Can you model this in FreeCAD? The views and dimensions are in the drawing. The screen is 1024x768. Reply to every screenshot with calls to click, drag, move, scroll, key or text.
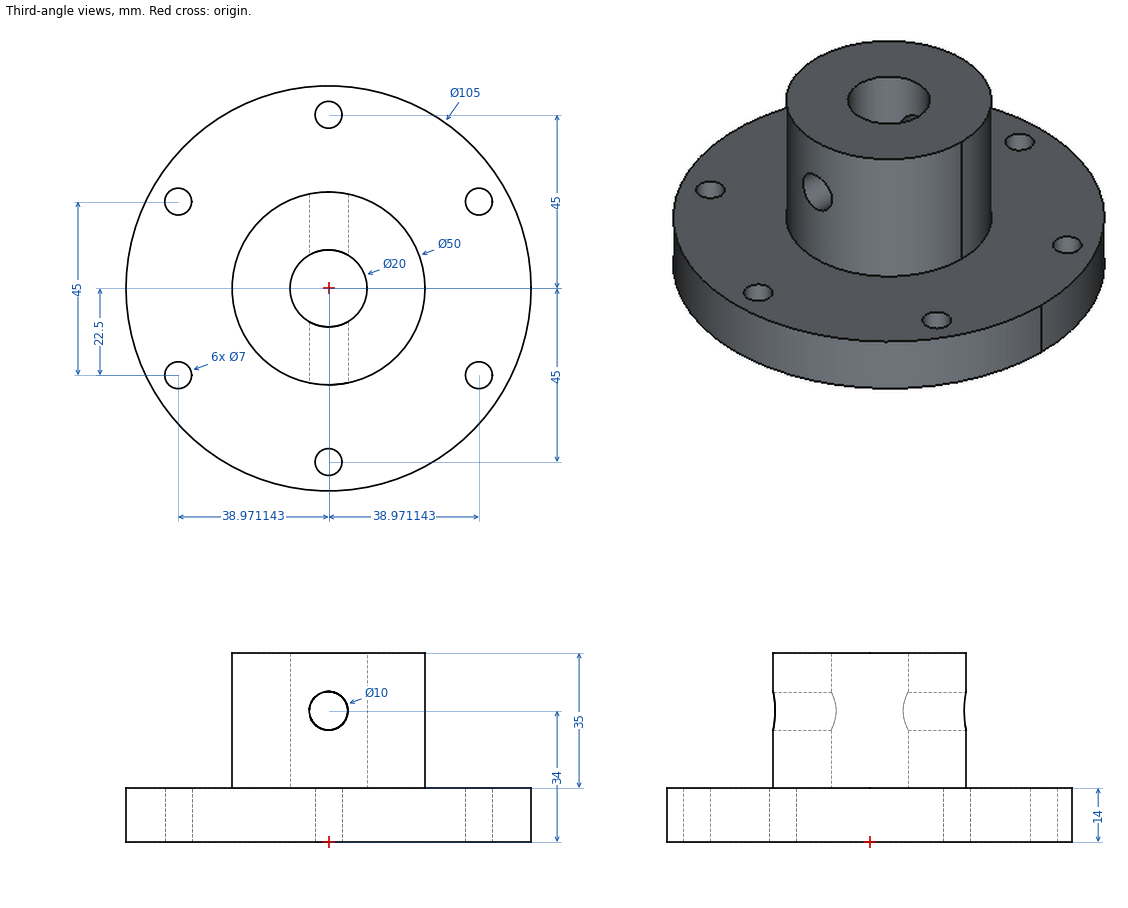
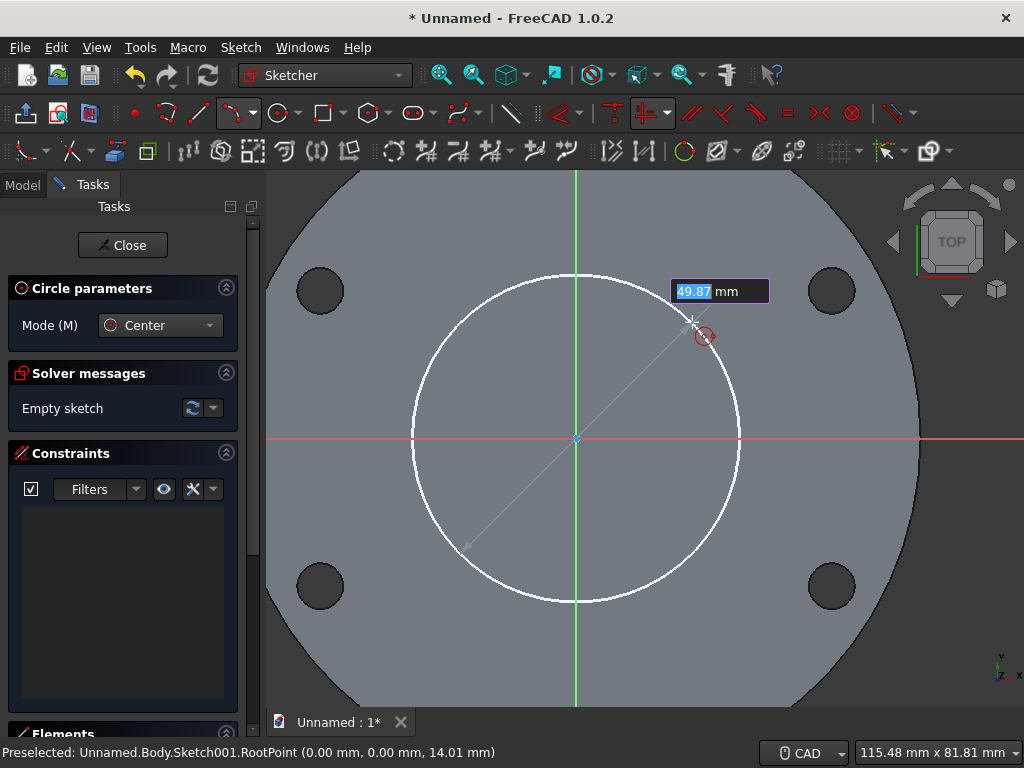
text(50)
key(Return)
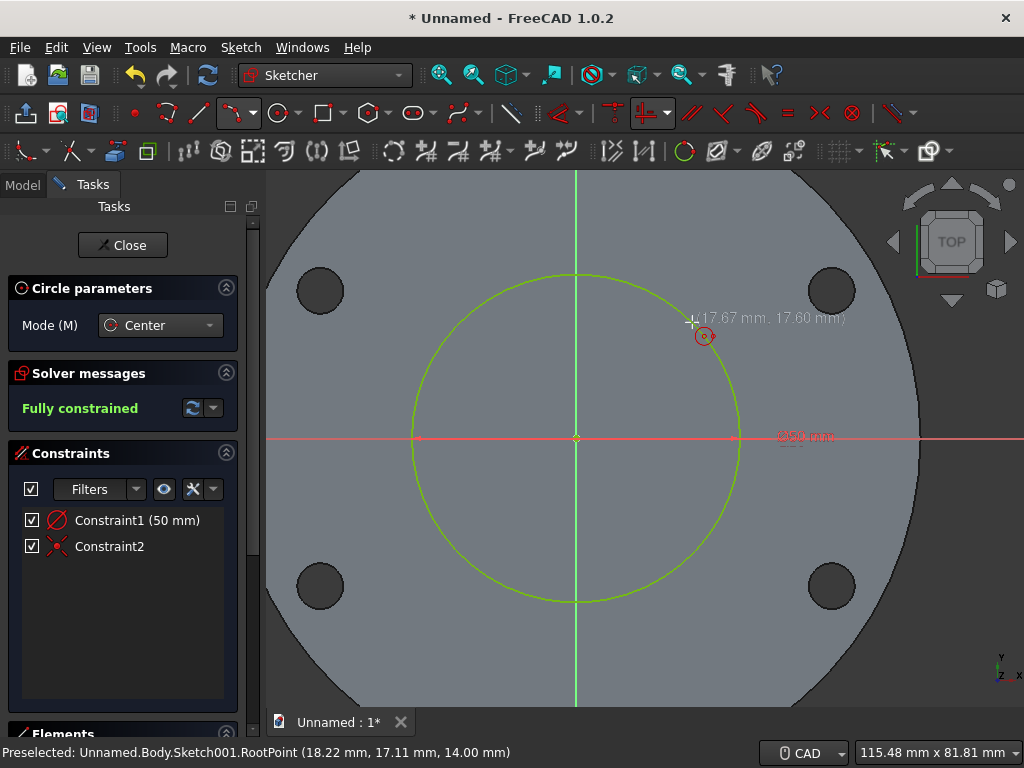
click(576, 438)
move(622, 392)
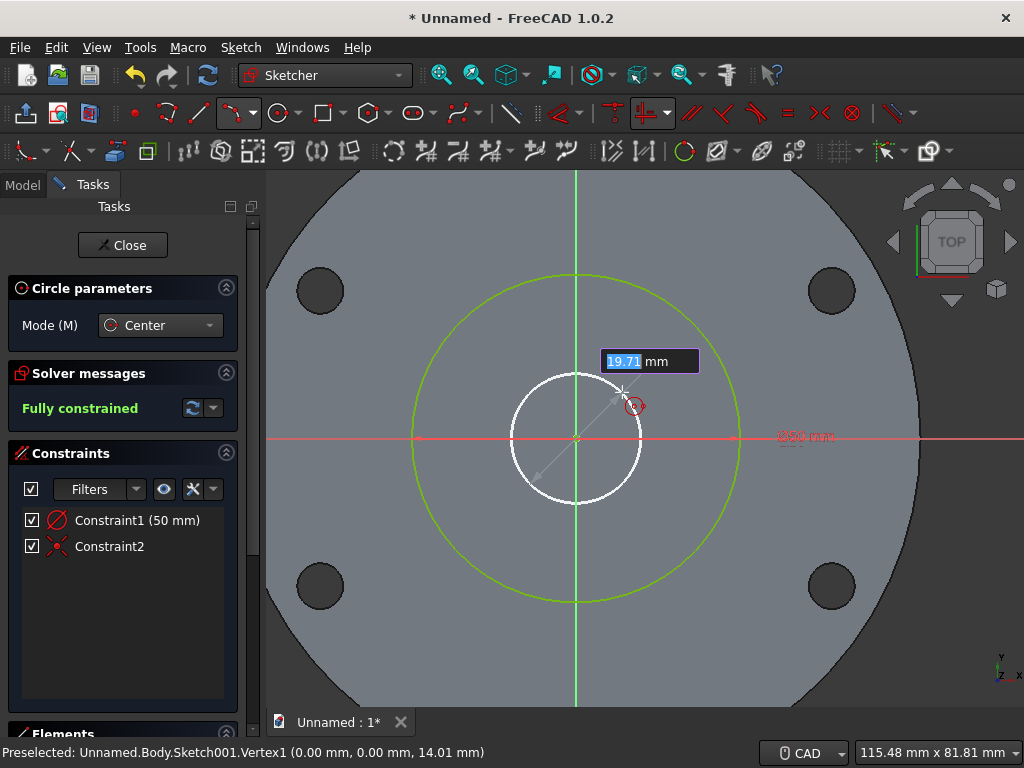
text(20)
key(Return)
key(Escape)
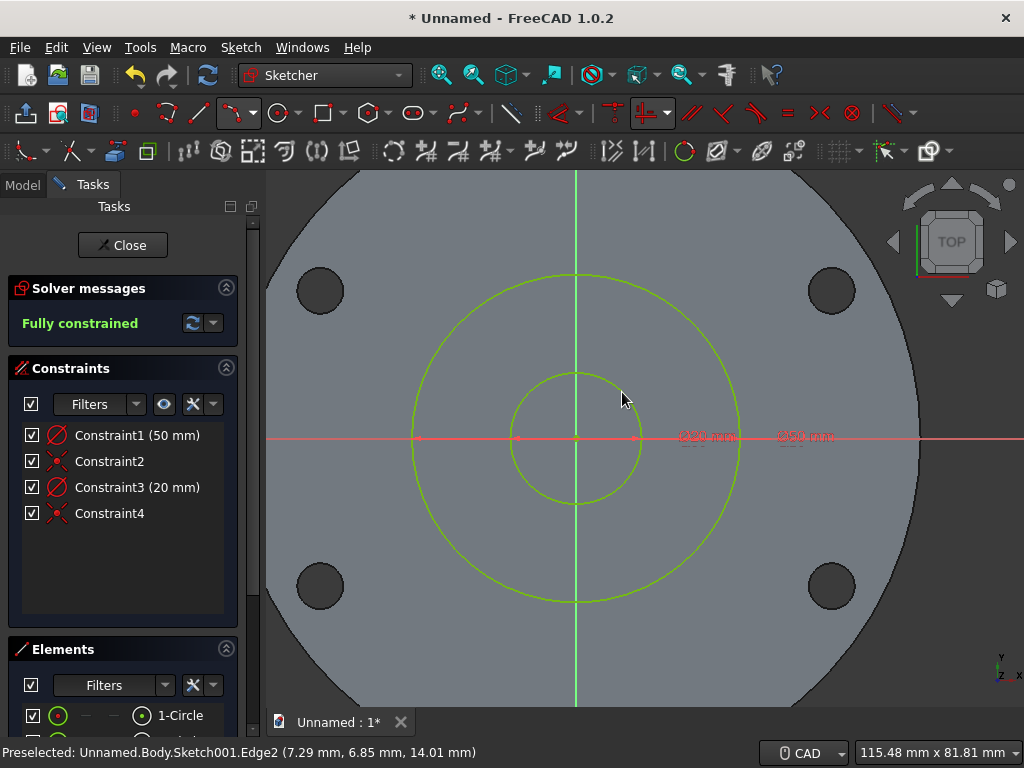
click(123, 245)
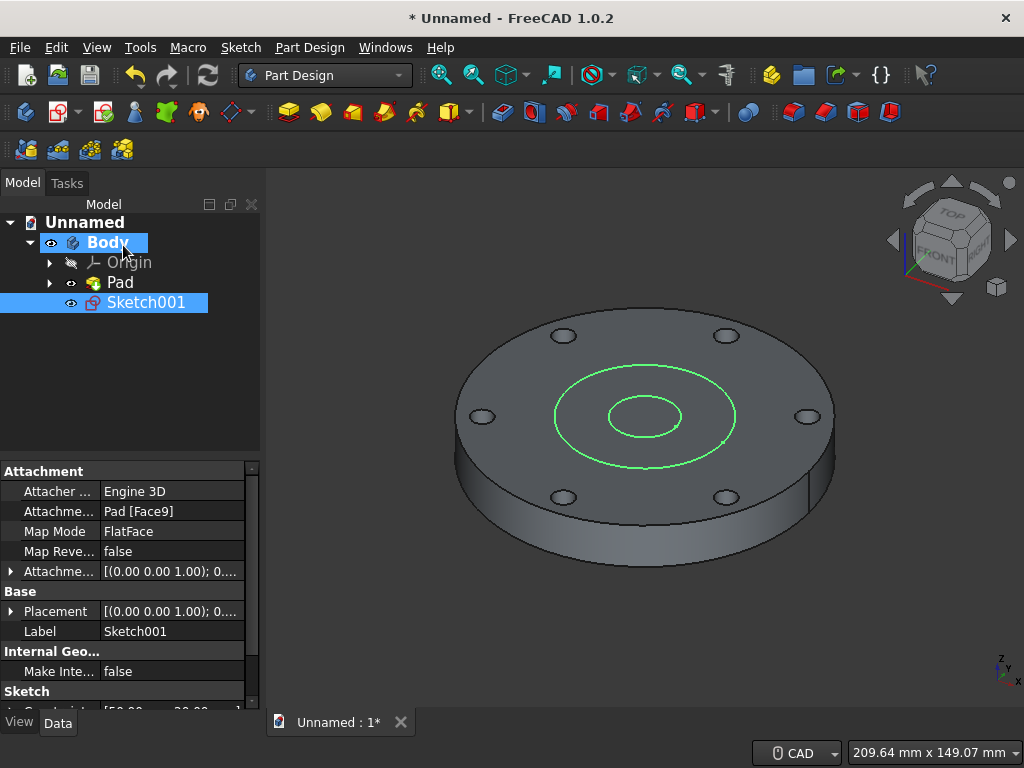
click(290, 112)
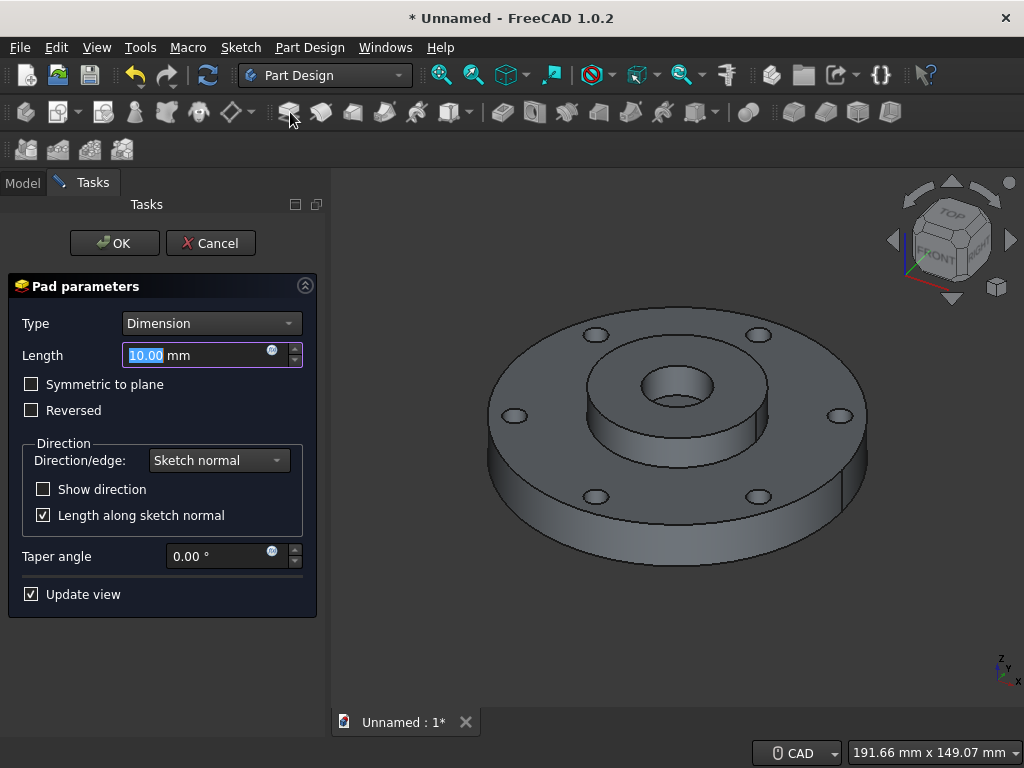
text(35)
key(Tab)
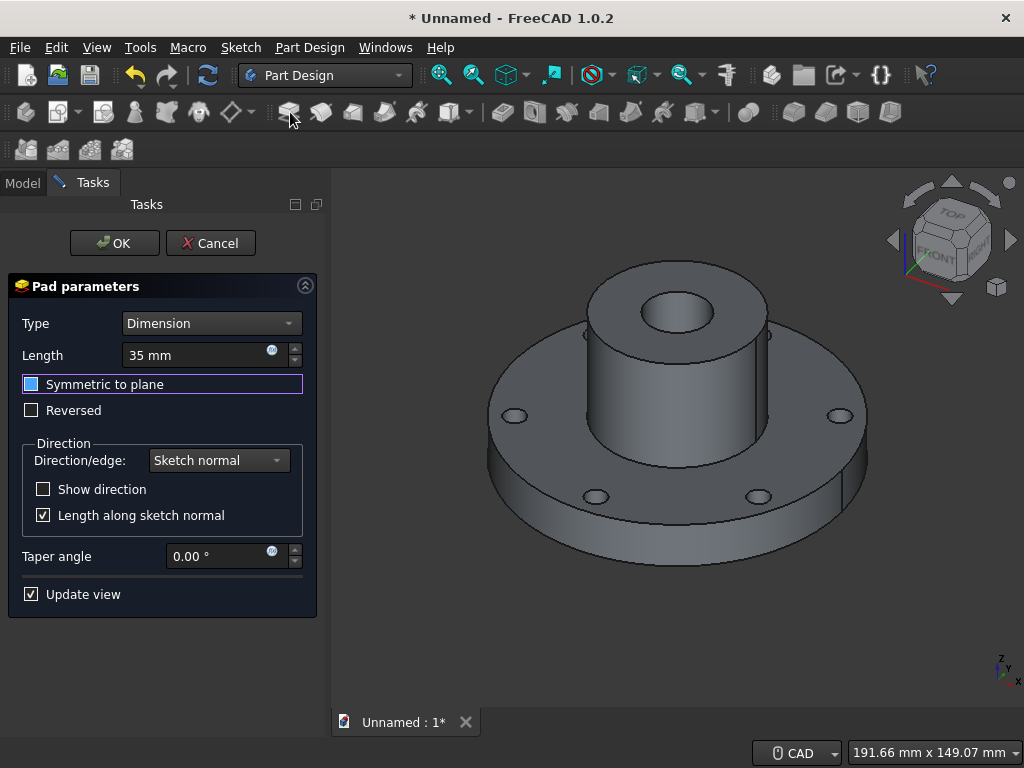
click(115, 243)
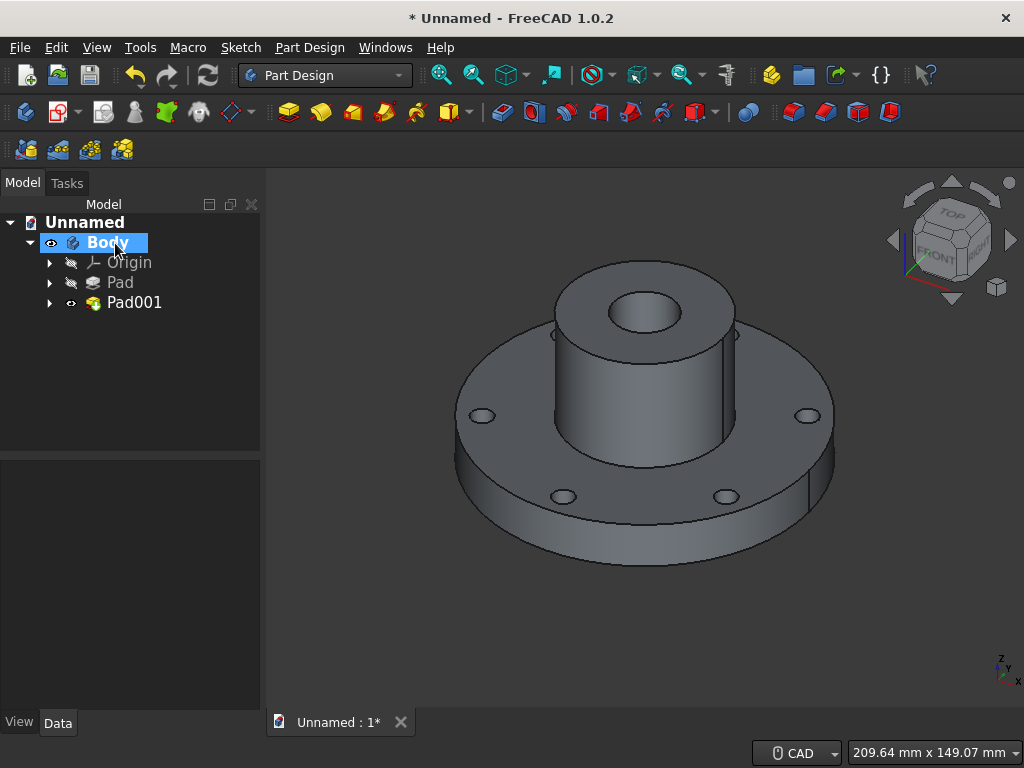
click(442, 76)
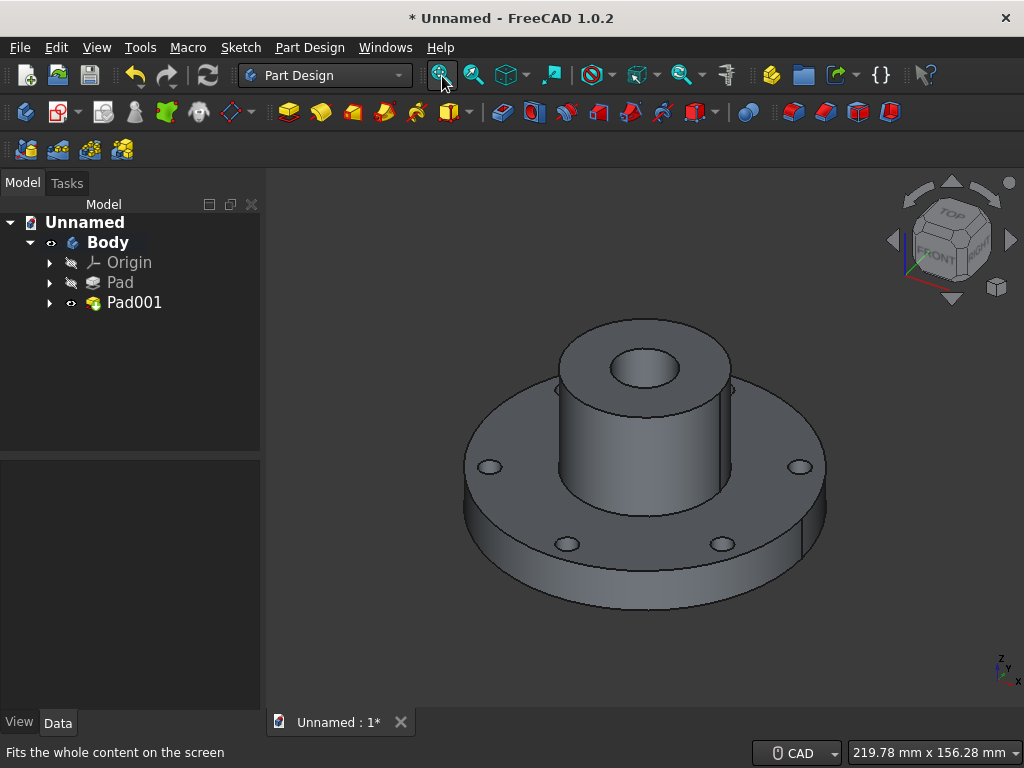
click(58, 112)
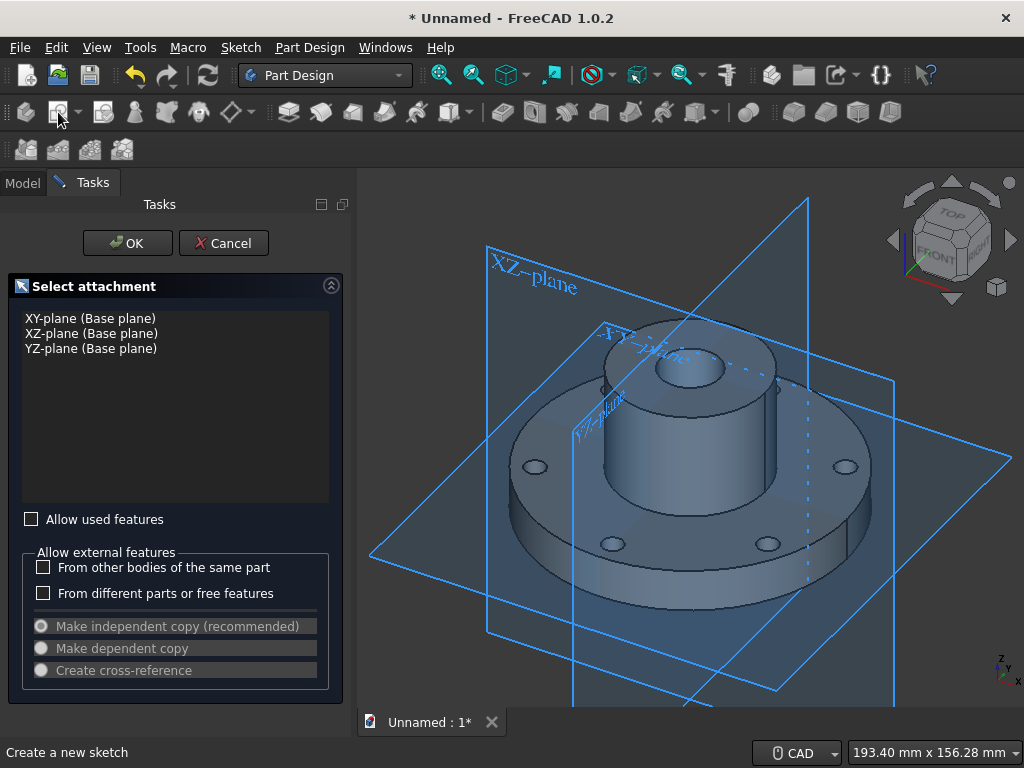
click(82, 334)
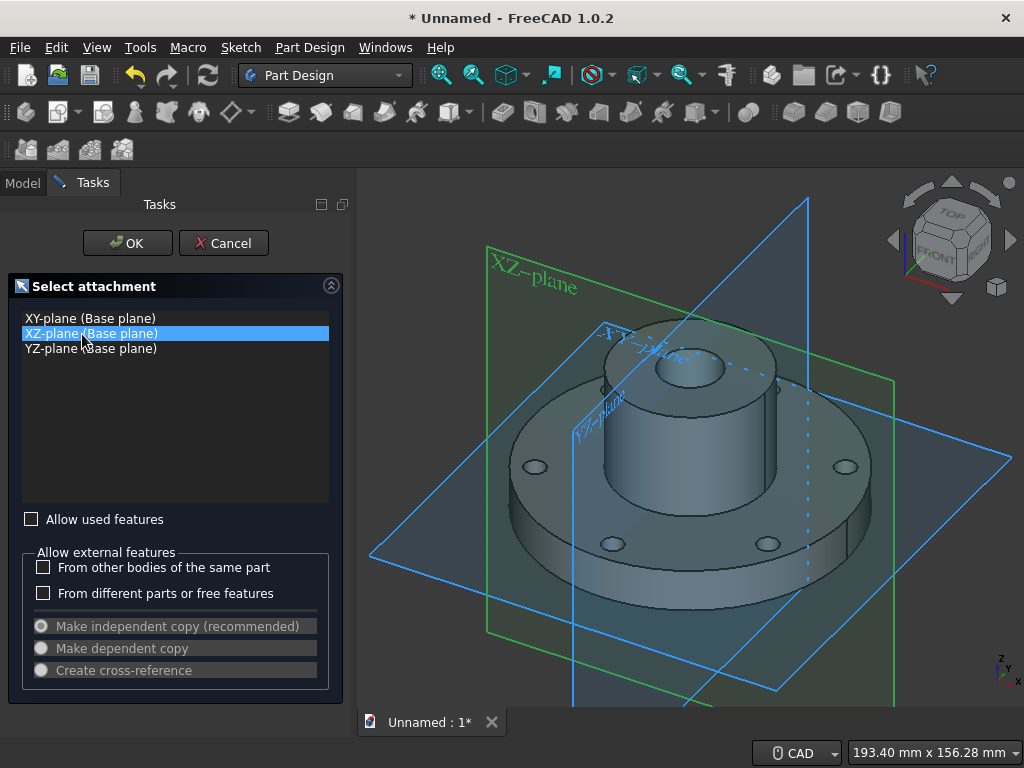
click(128, 243)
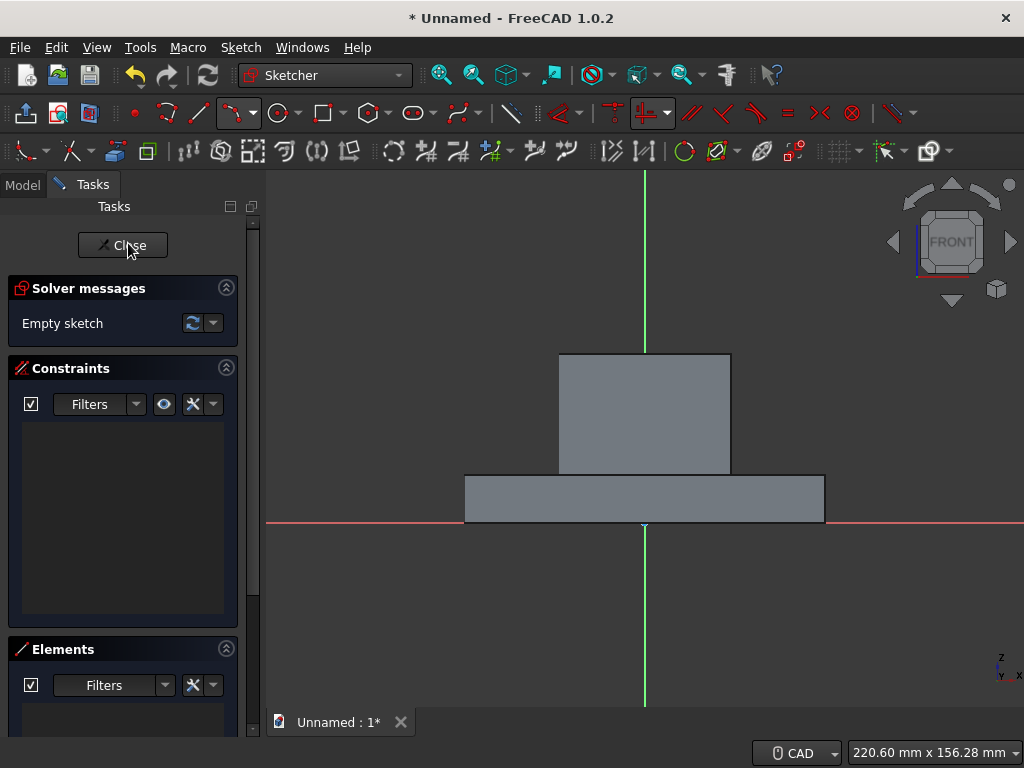
key(q)
key(s)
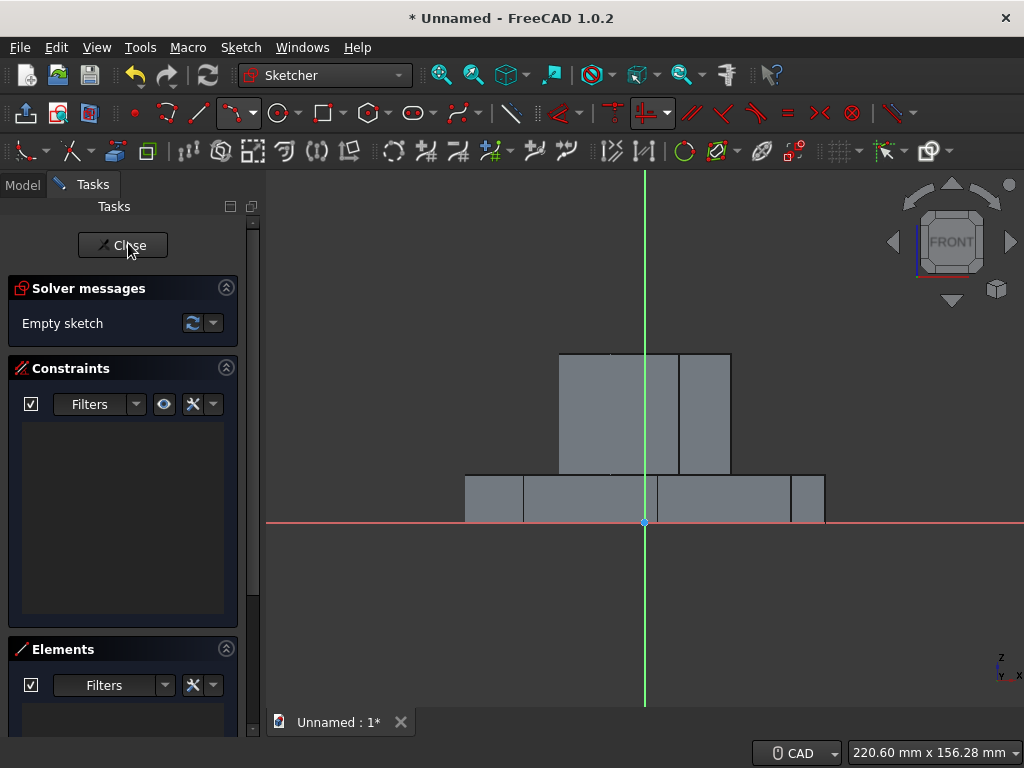
scroll(653, 402, up, 11)